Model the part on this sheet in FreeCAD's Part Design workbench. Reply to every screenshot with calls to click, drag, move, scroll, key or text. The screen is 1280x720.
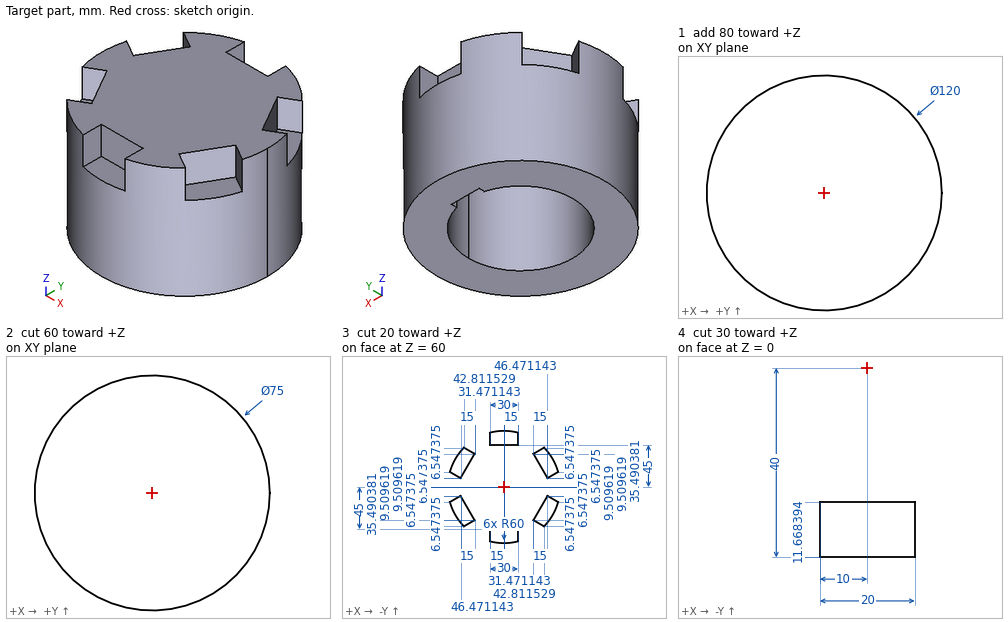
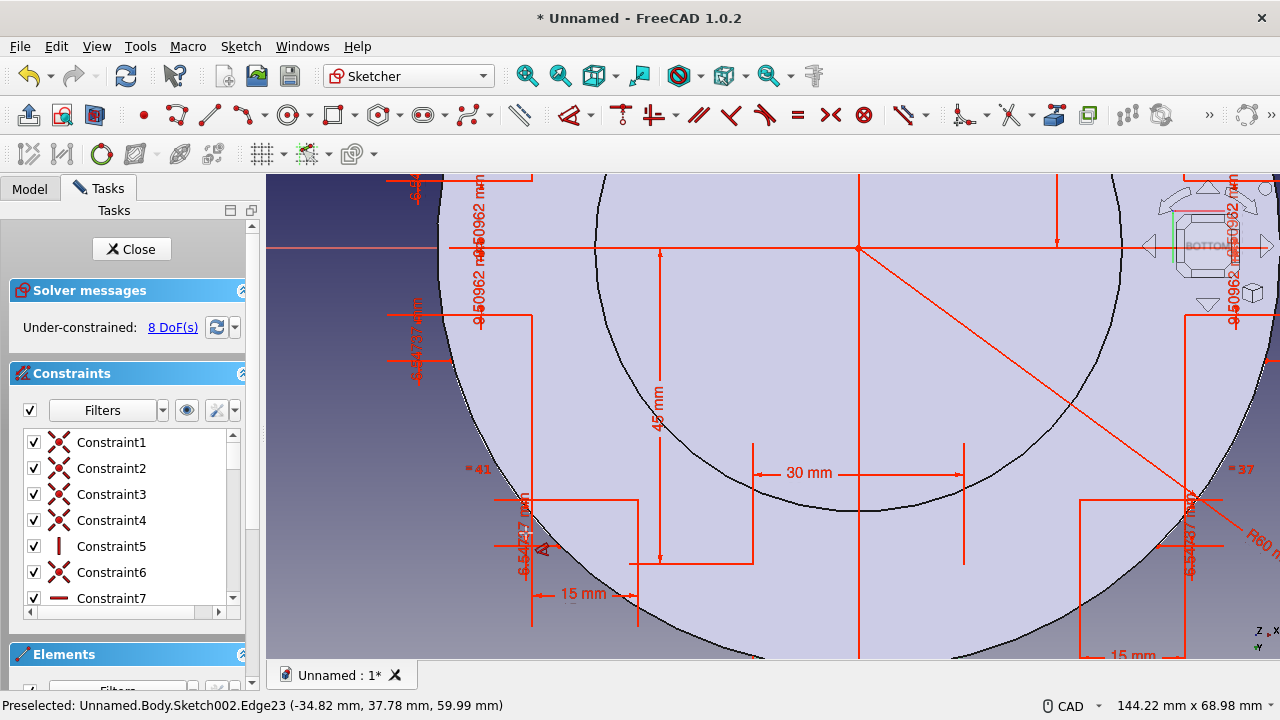
scroll(615, 515, down, 5)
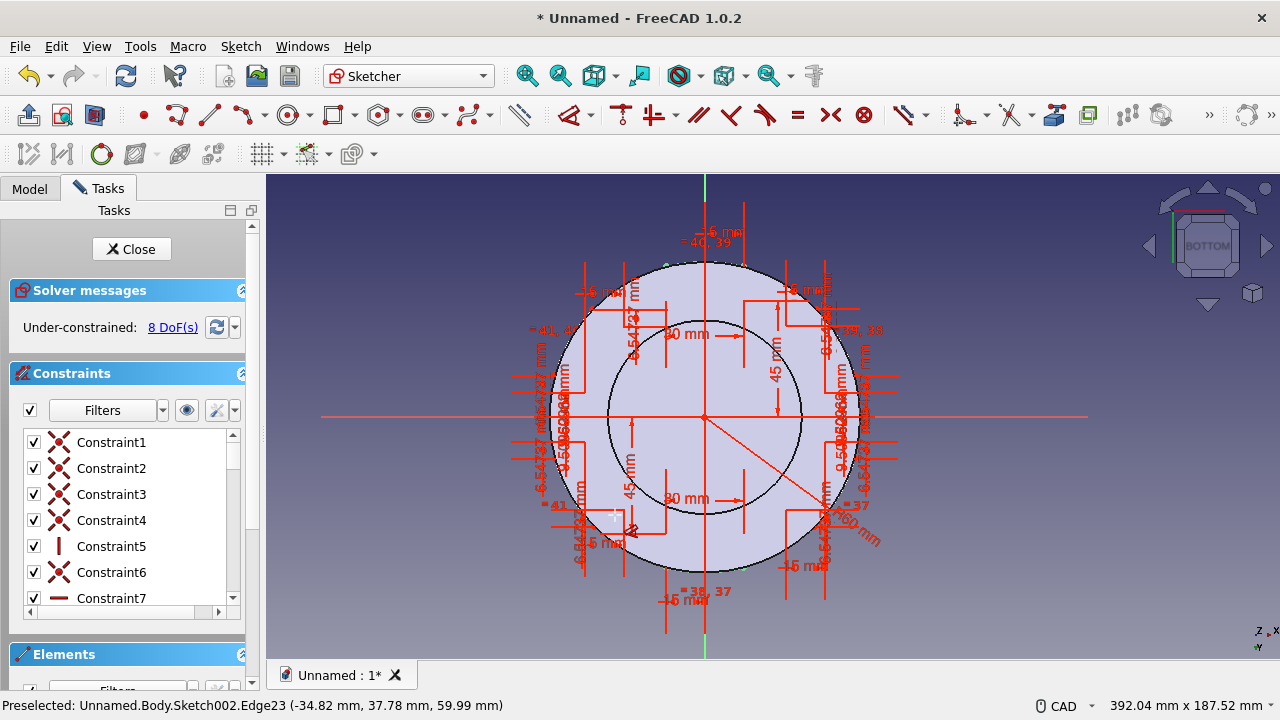
click(815, 527)
click(760, 383)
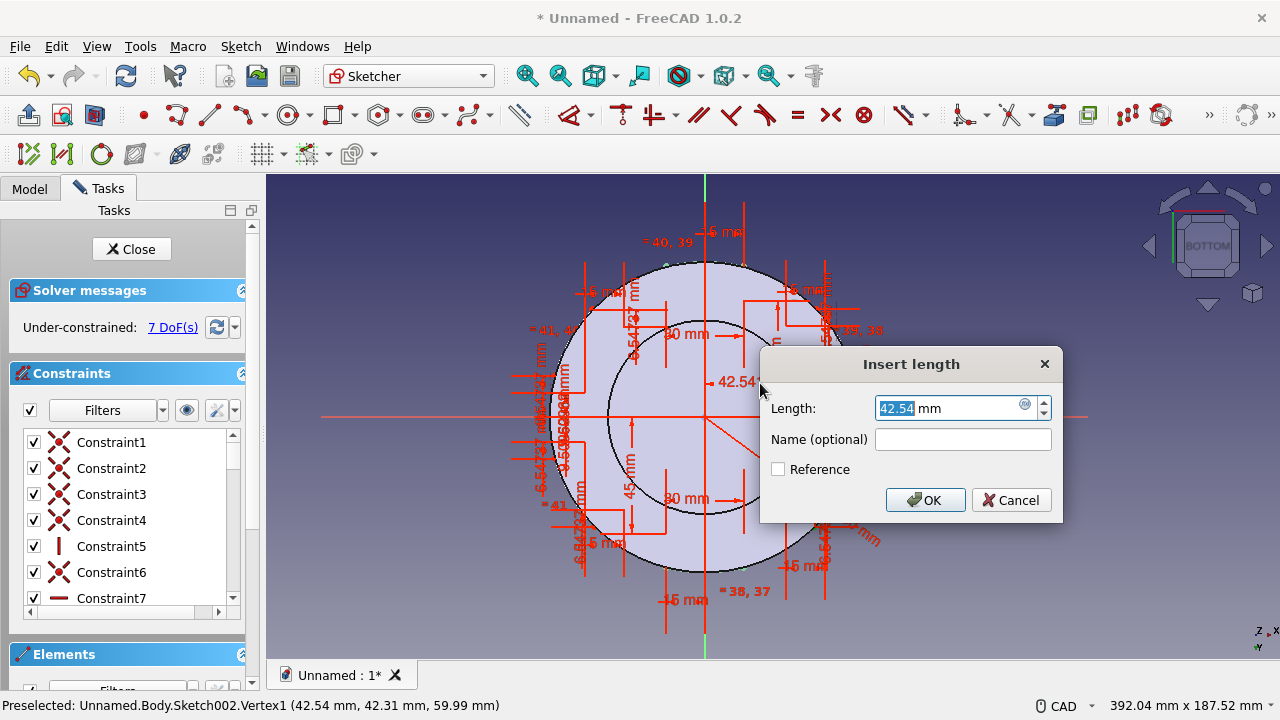
text(42.811529)
key(Return)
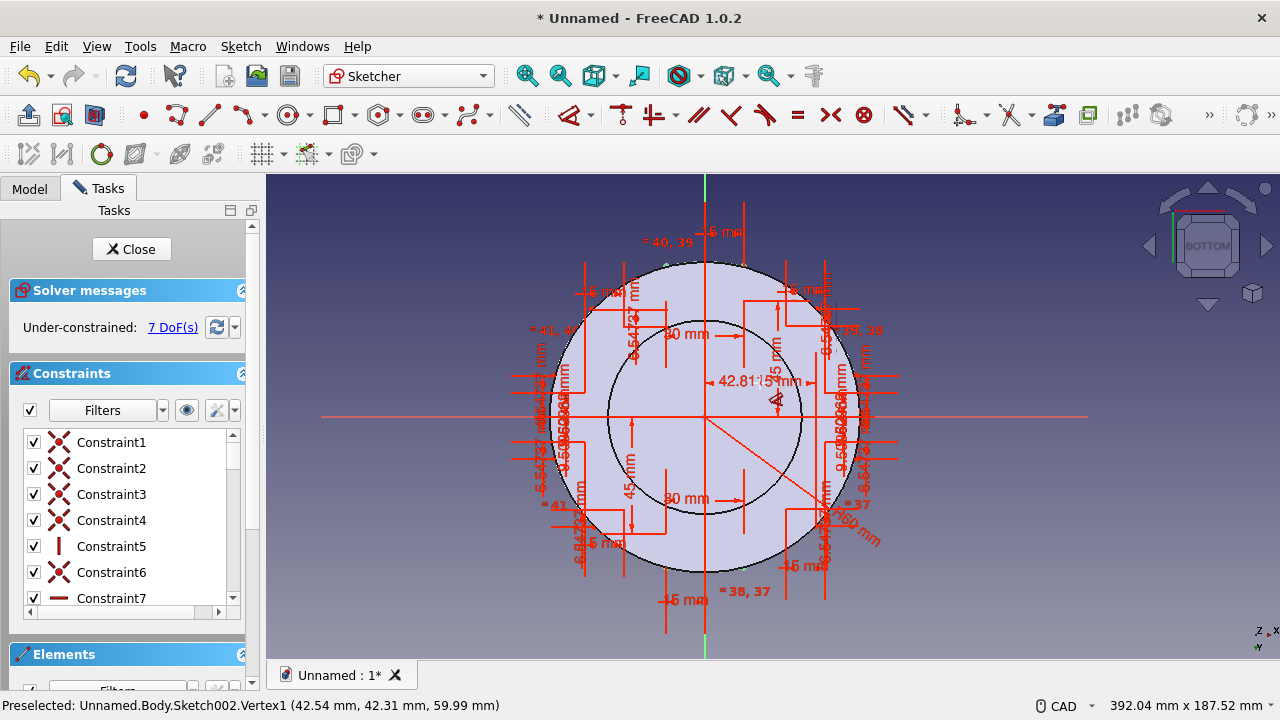
click(786, 509)
click(764, 543)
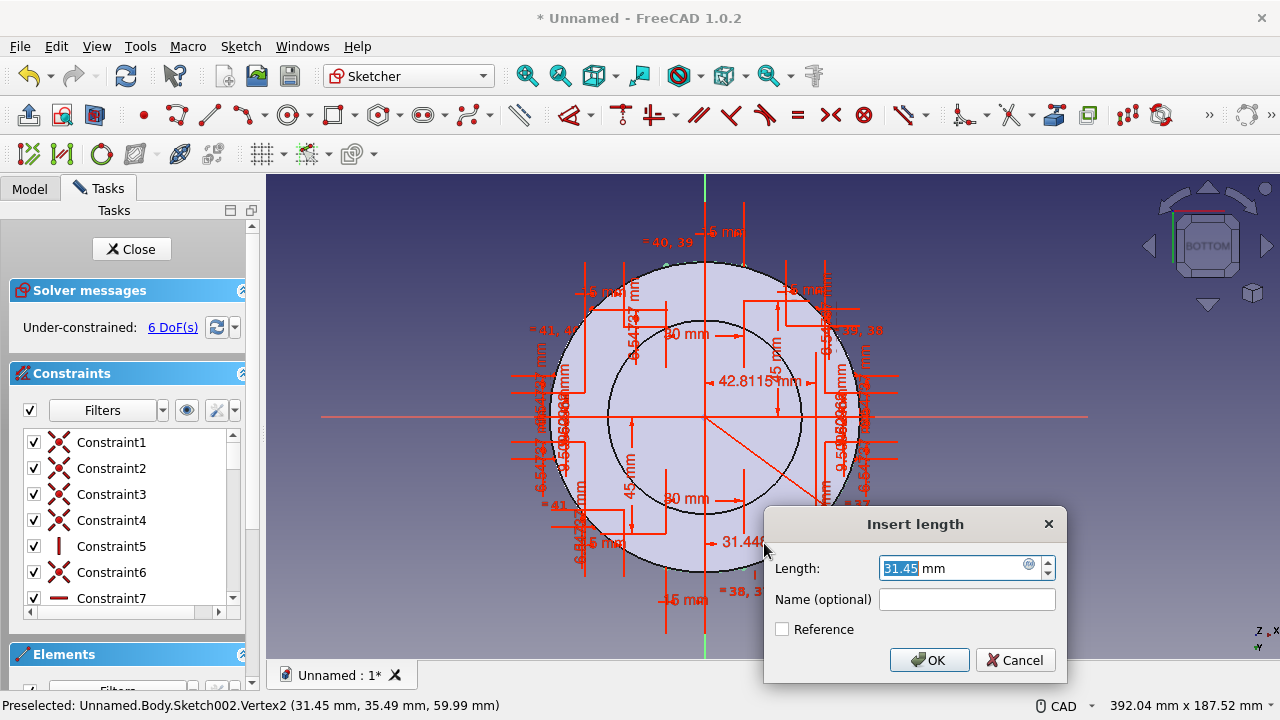
text(31.471143)
key(Return)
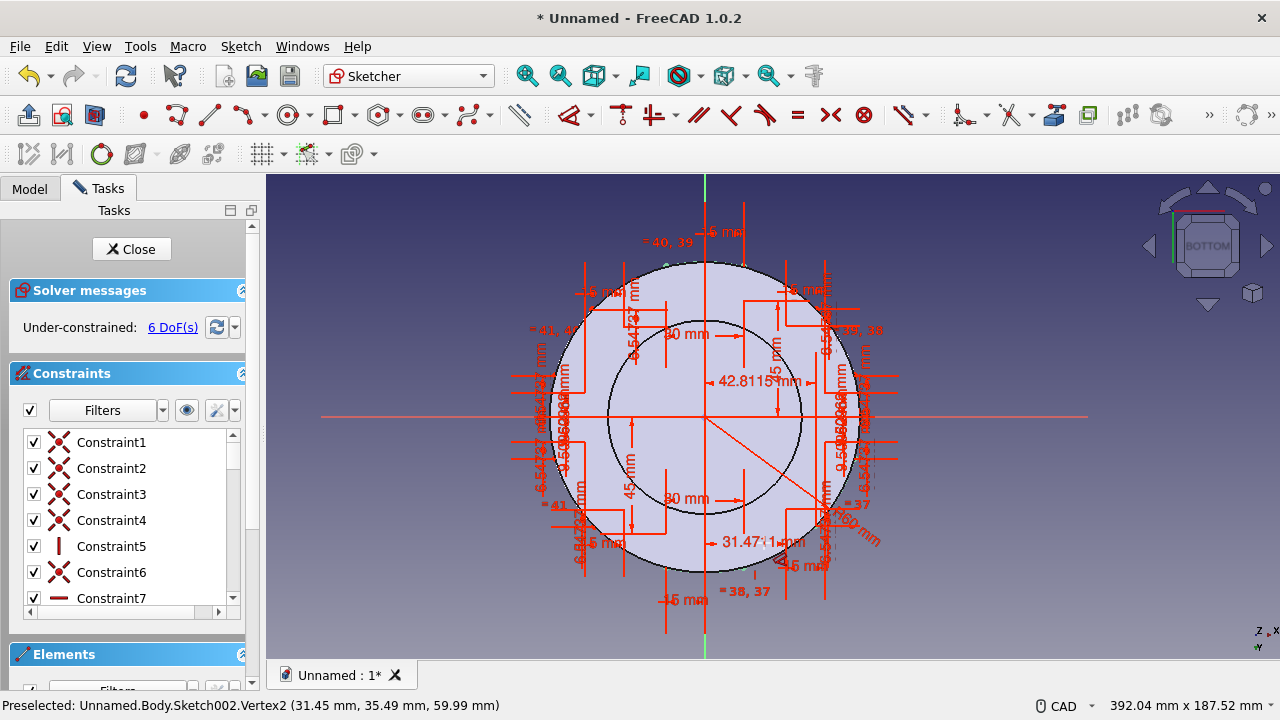
click(825, 393)
click(765, 451)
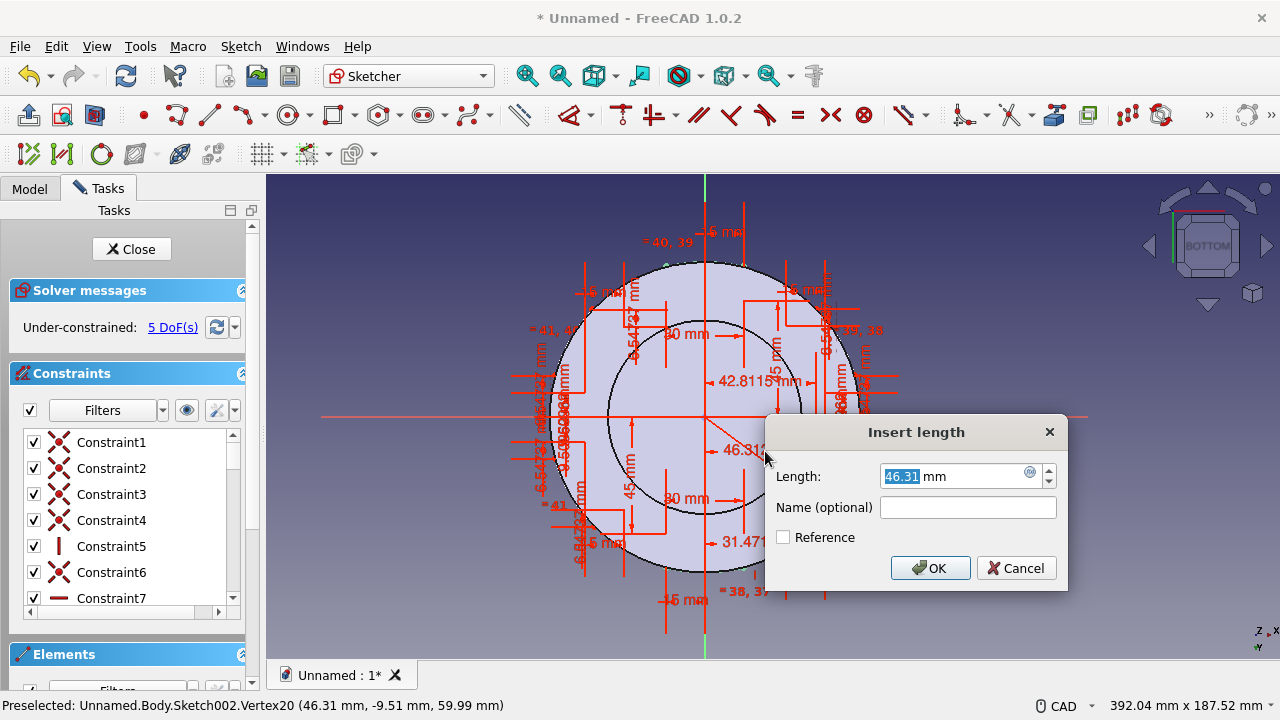
text(46.471143)
key(Return)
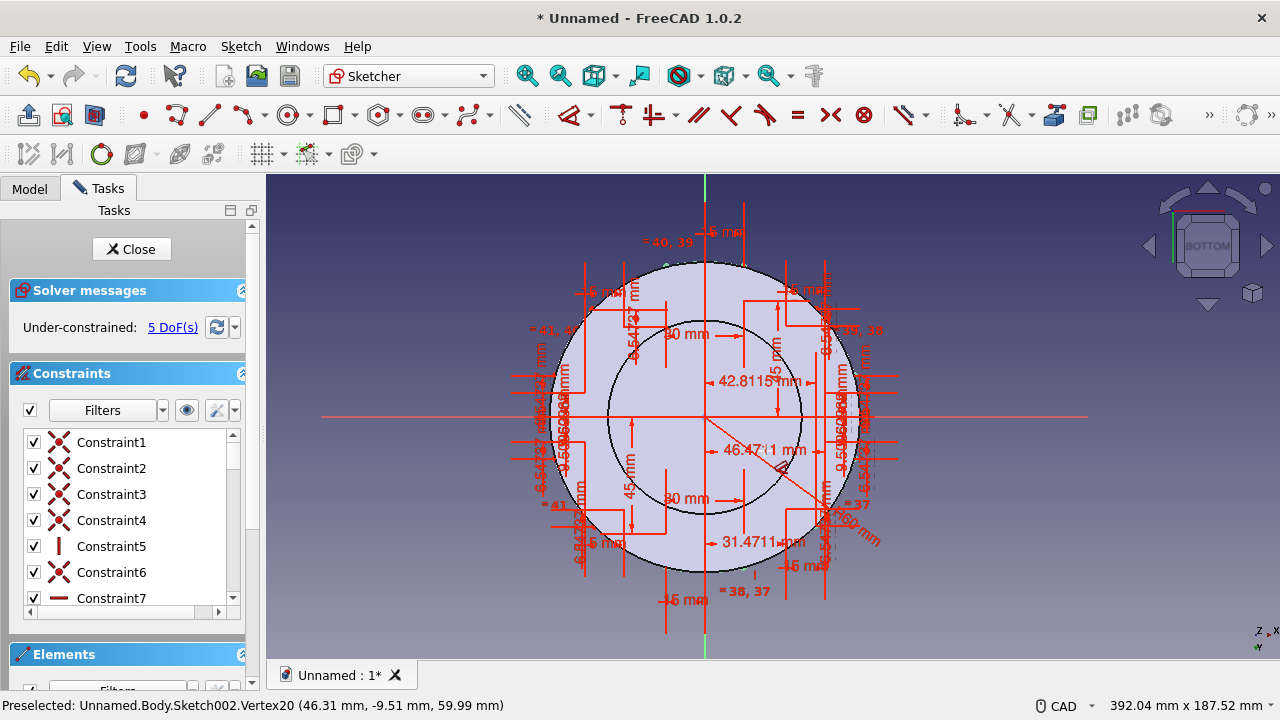
click(786, 326)
click(671, 372)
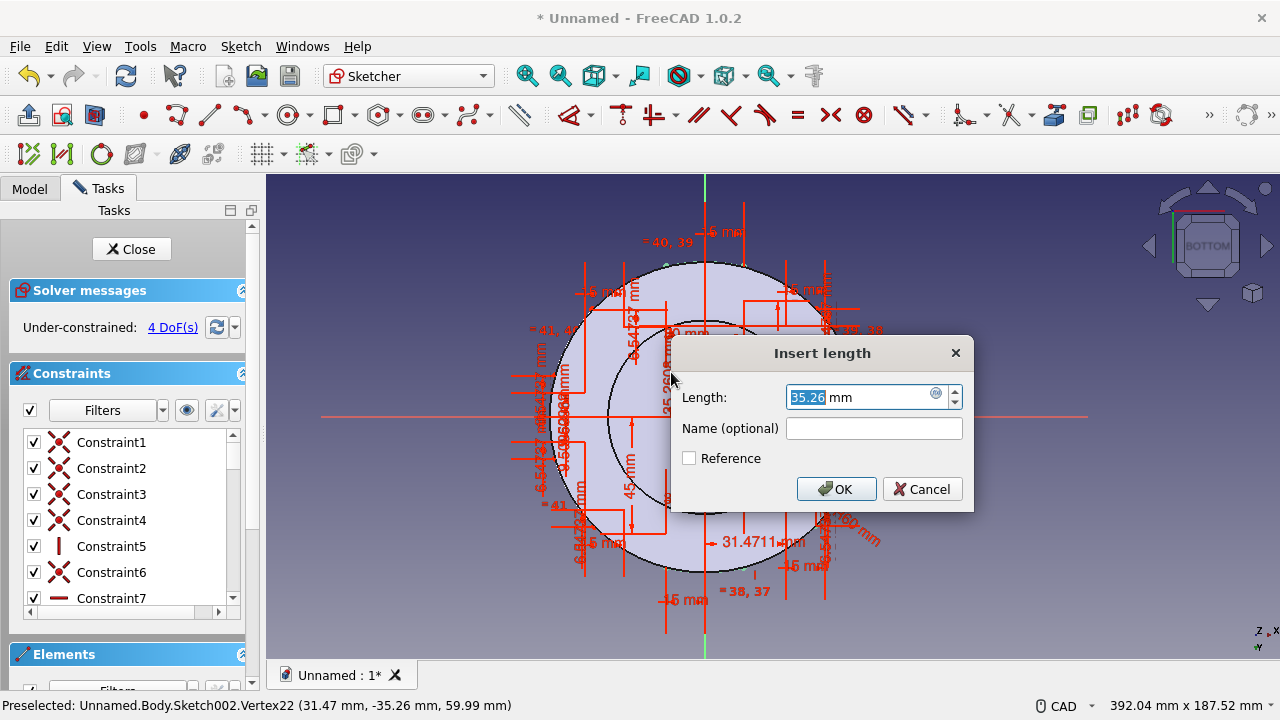
text(35.490381)
key(Return)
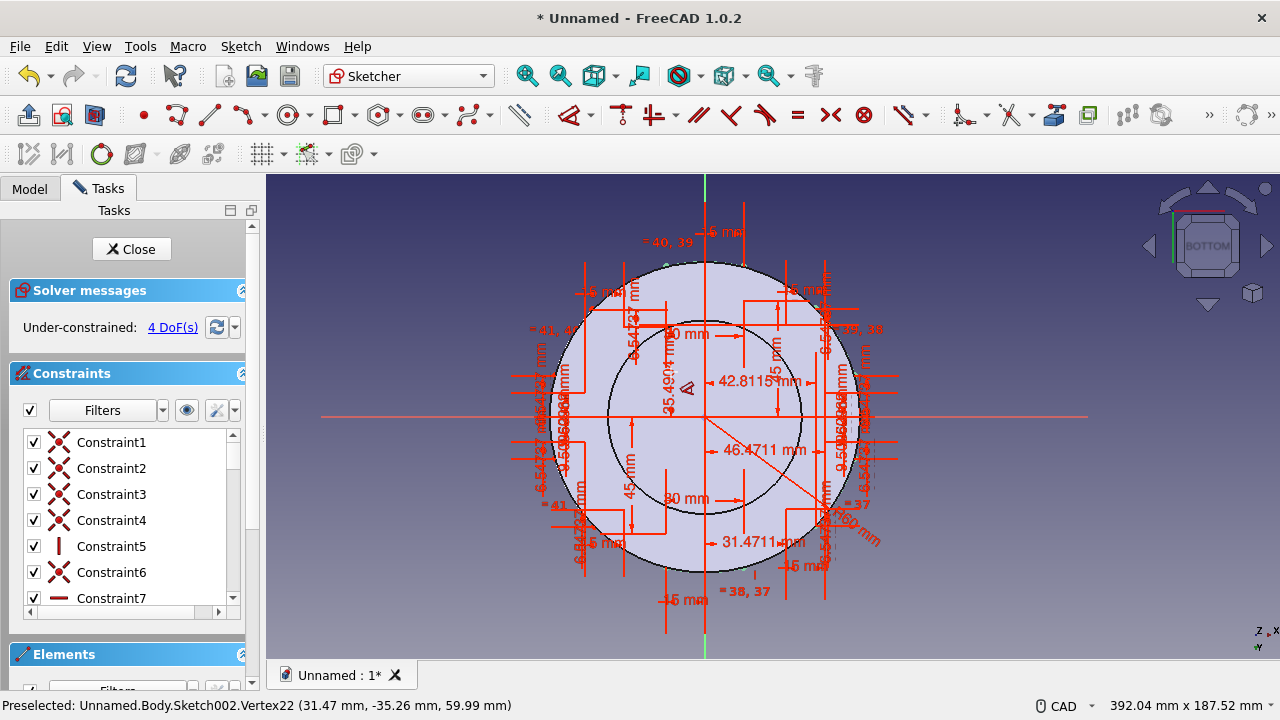
click(593, 310)
click(649, 451)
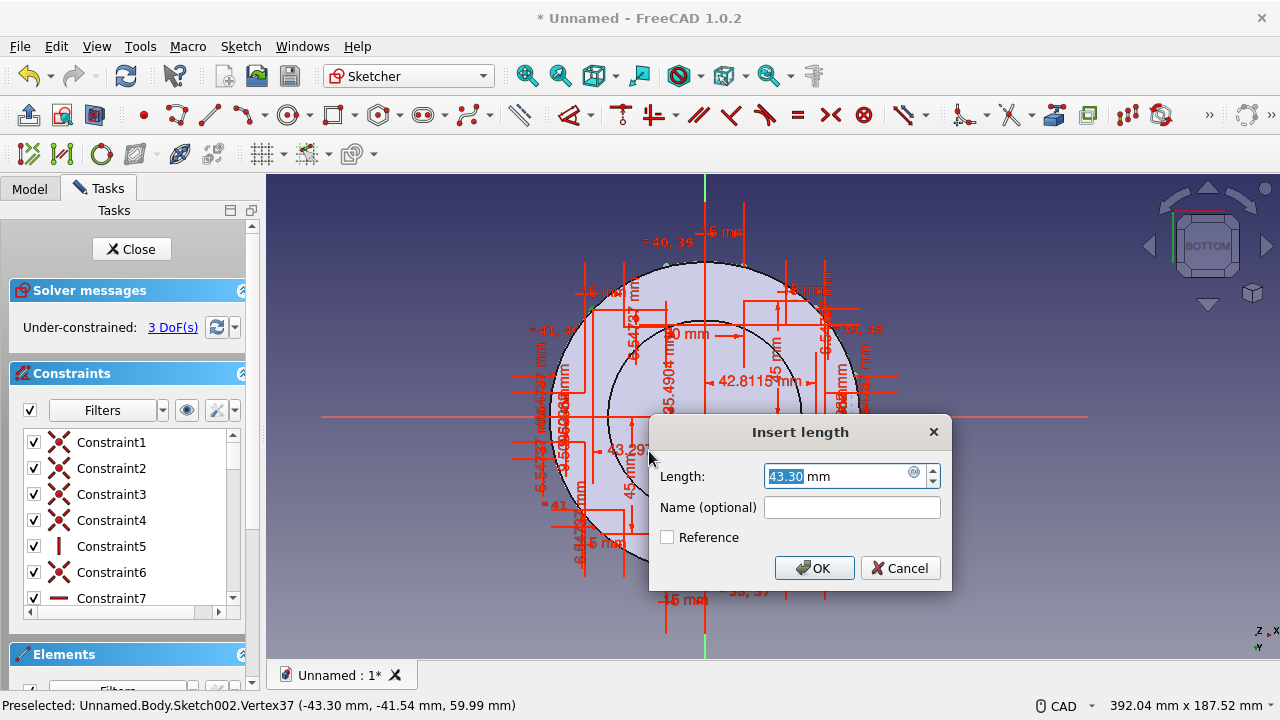
text(42.811529)
key(Return)